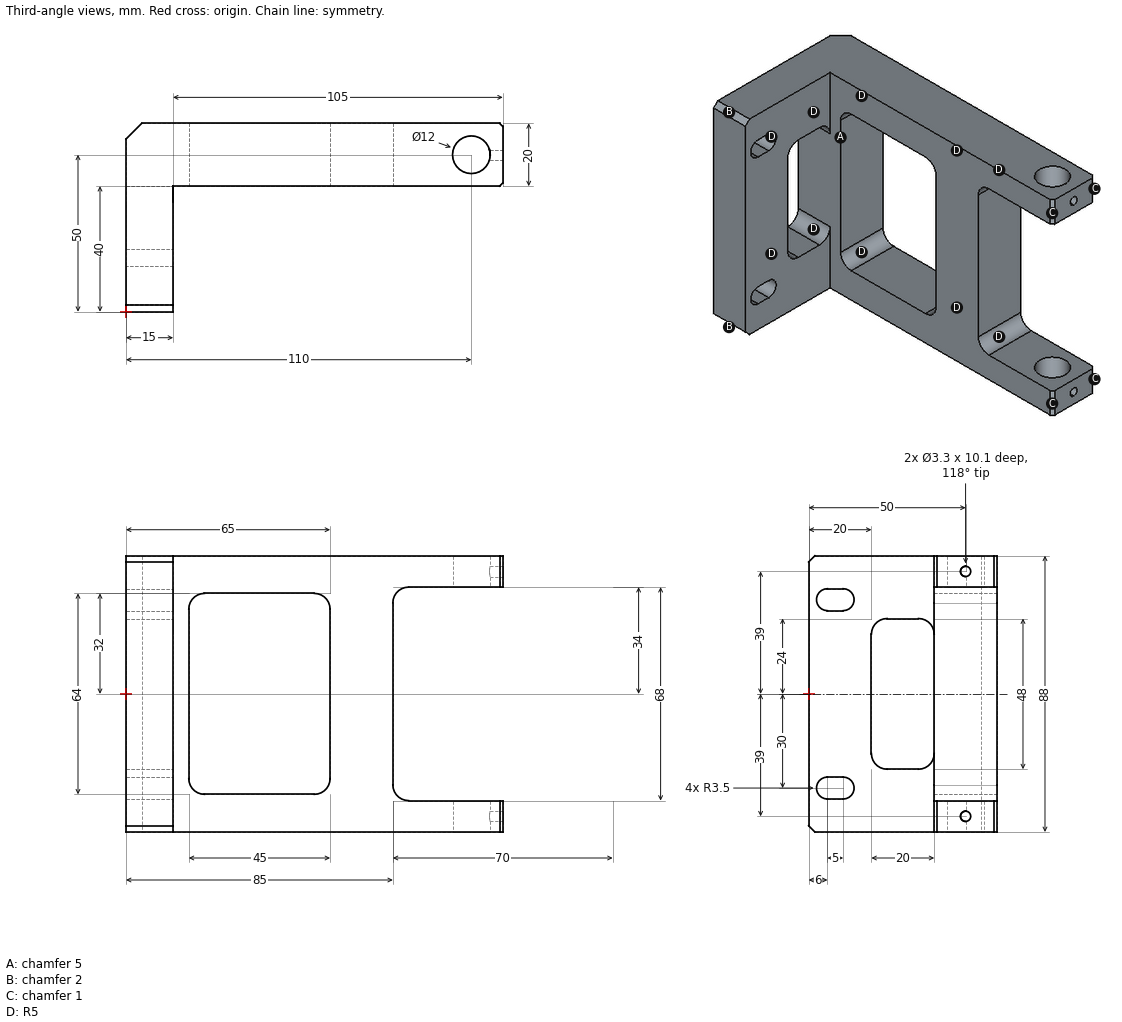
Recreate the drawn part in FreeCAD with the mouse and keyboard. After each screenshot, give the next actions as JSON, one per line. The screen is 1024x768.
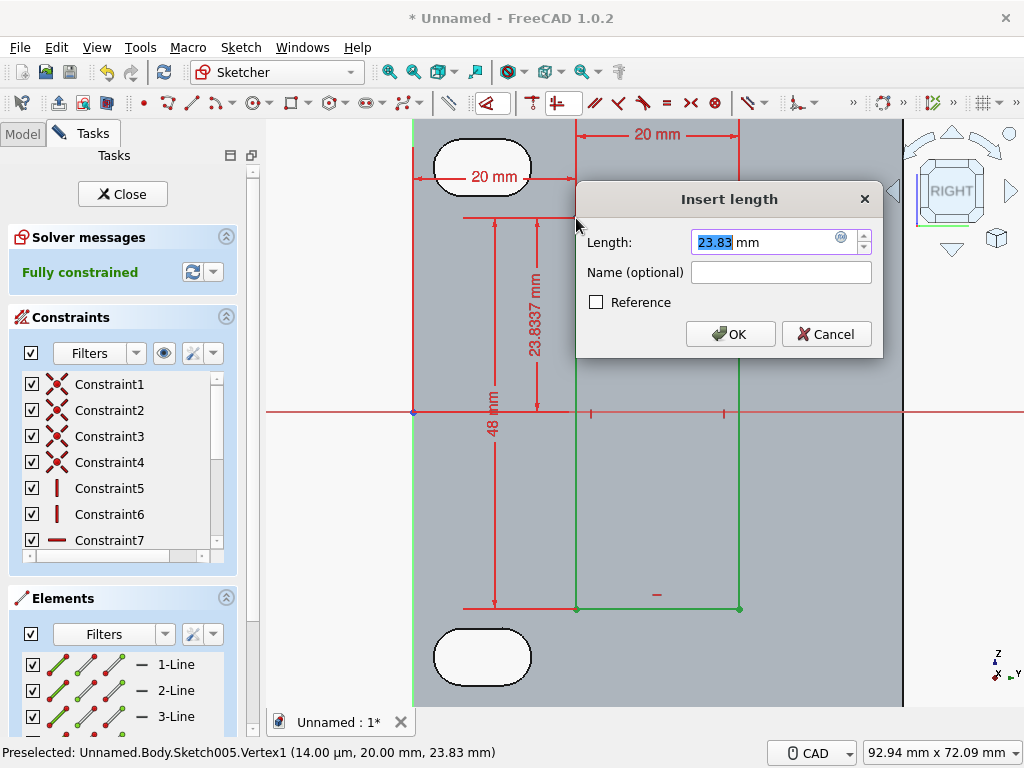
{"action": "type", "text": "24"}
{"action": "key", "text": "Return"}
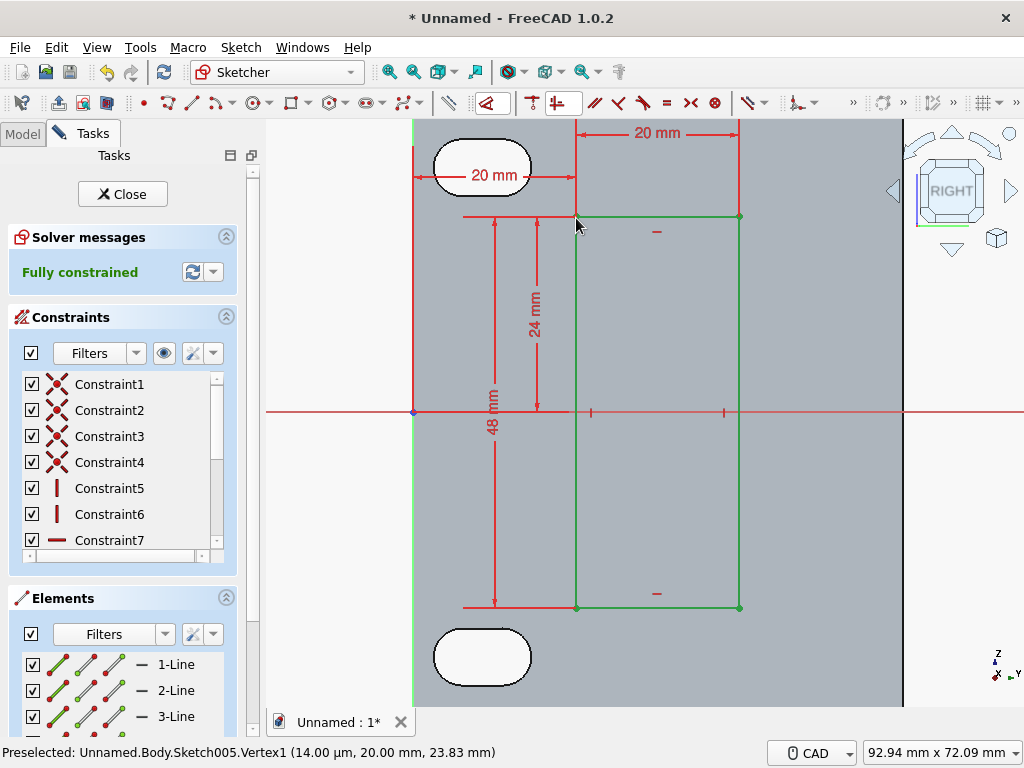
{"action": "left_click", "coordinate": [123, 194]}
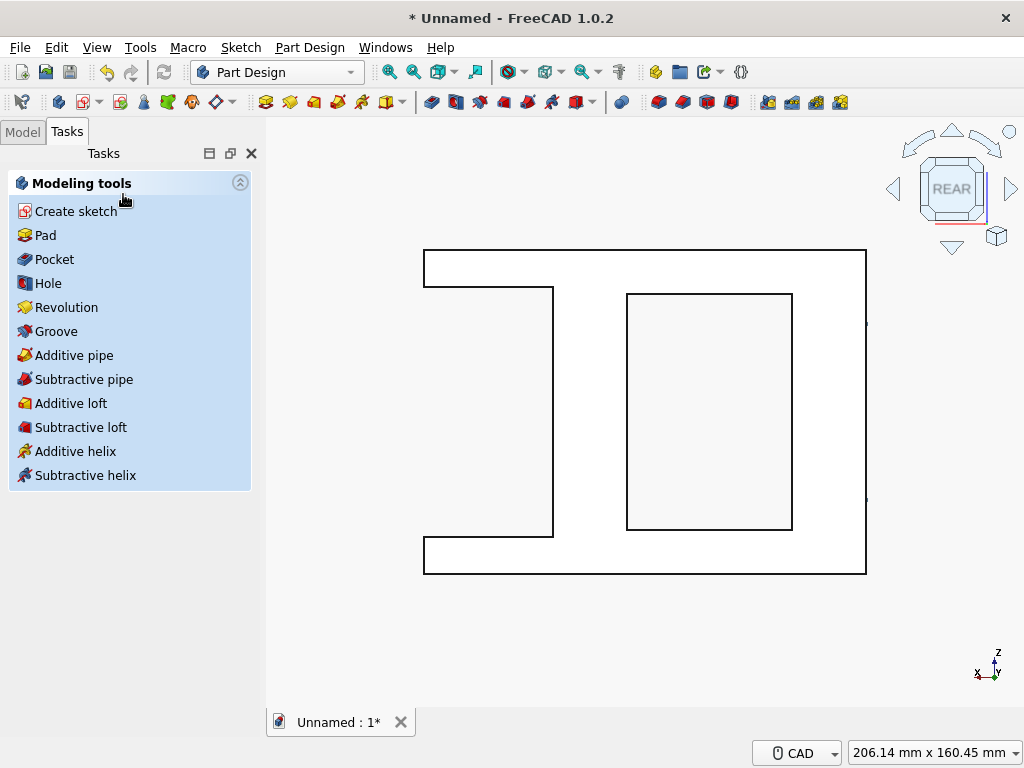
{"action": "left_click", "coordinate": [432, 102]}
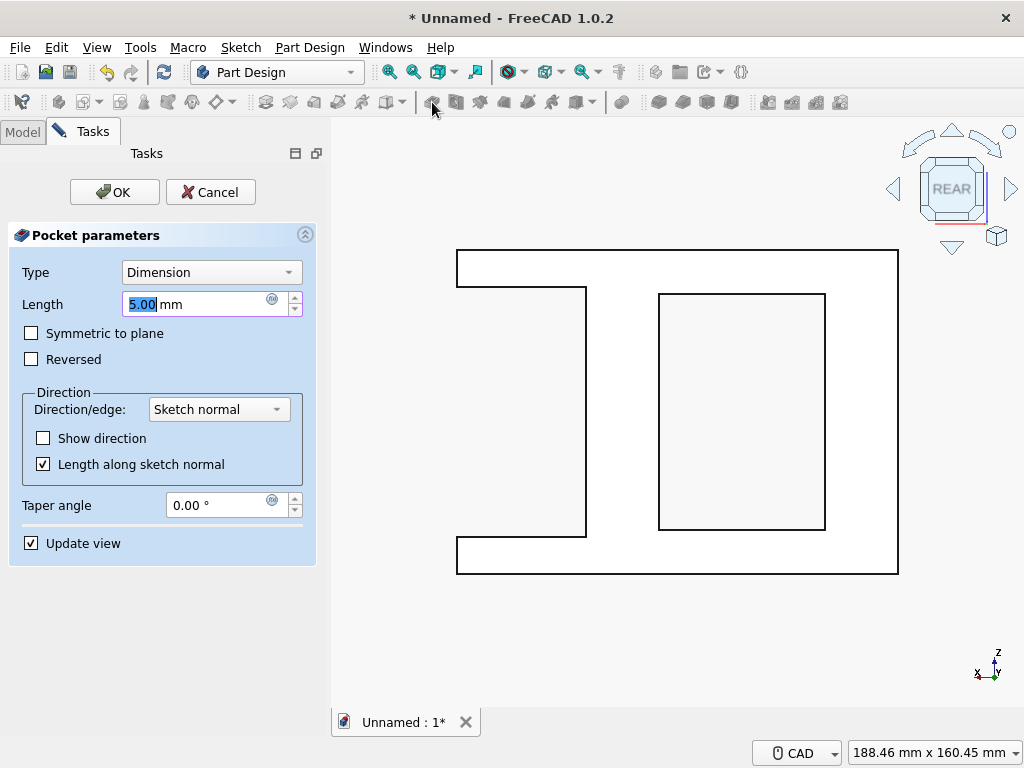
{"action": "left_click", "coordinate": [212, 272]}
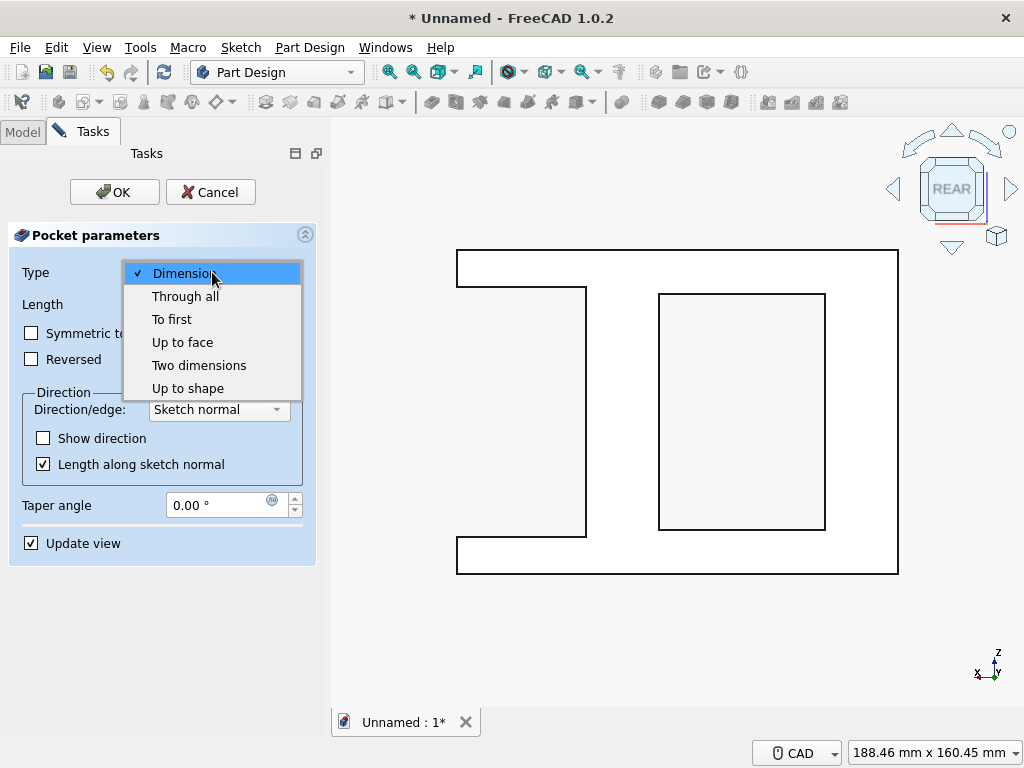
{"action": "left_click", "coordinate": [212, 296]}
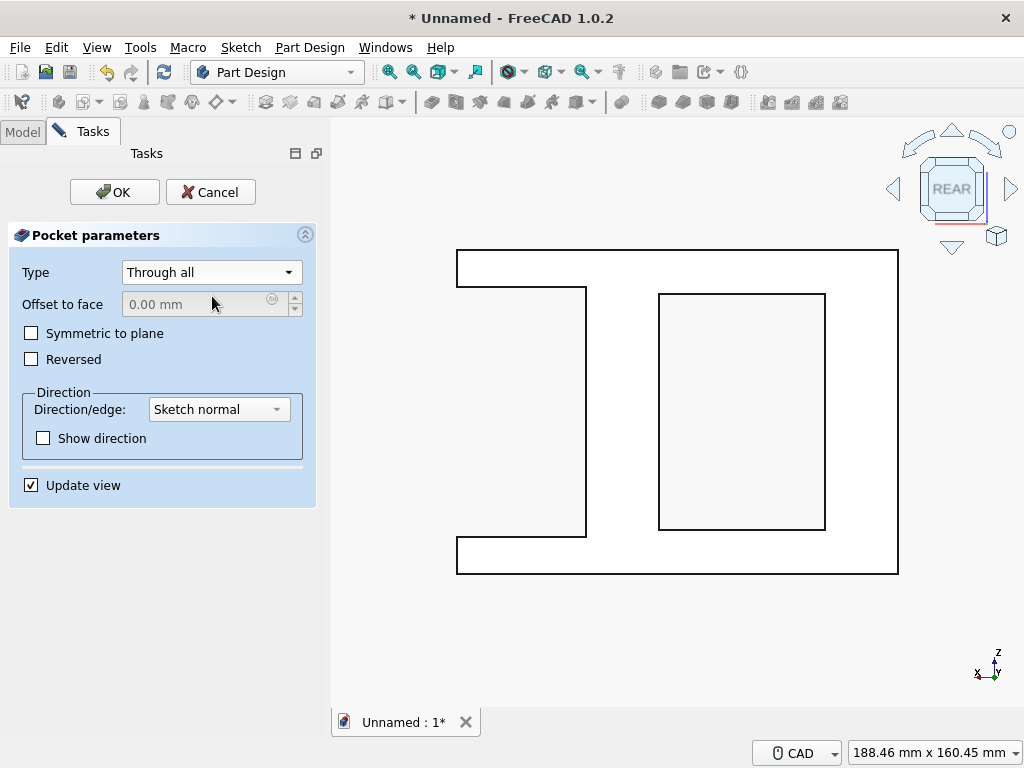
{"action": "left_click", "coordinate": [30, 359]}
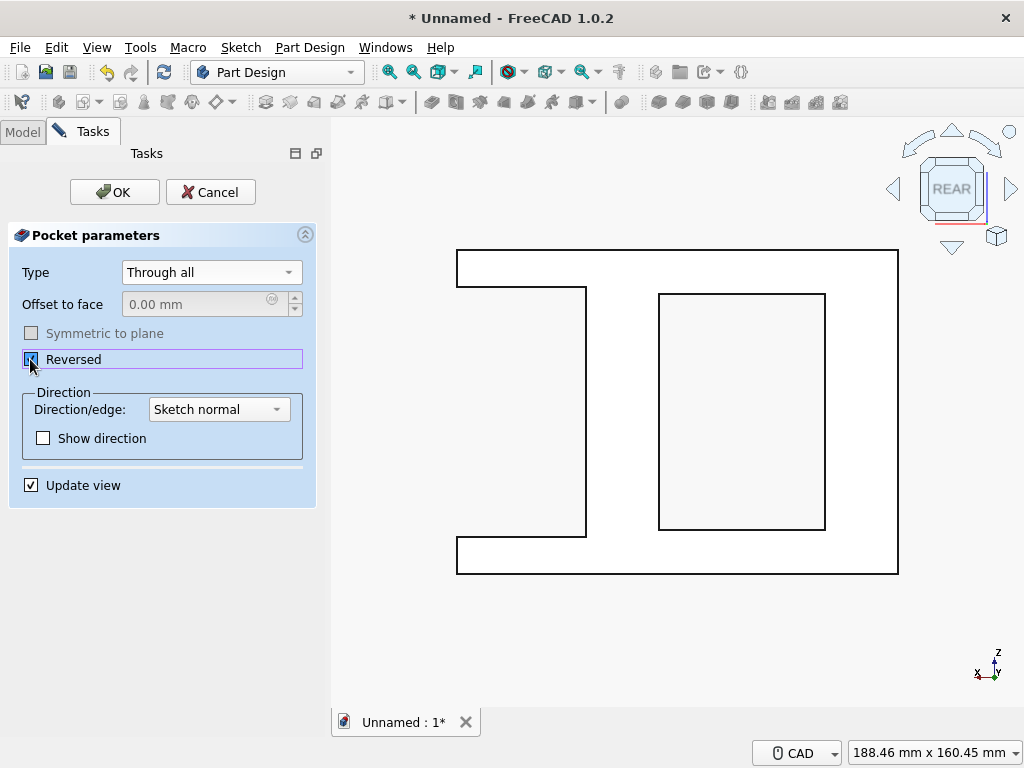
{"action": "left_click", "coordinate": [115, 192]}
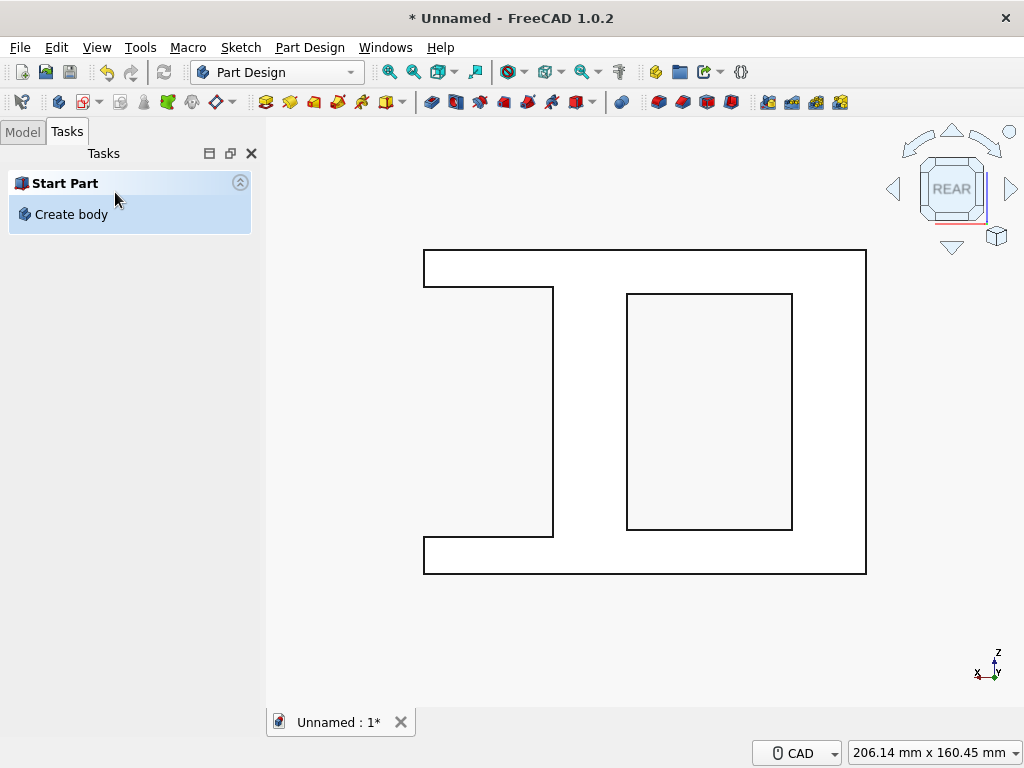
{"action": "left_click", "coordinate": [866, 411]}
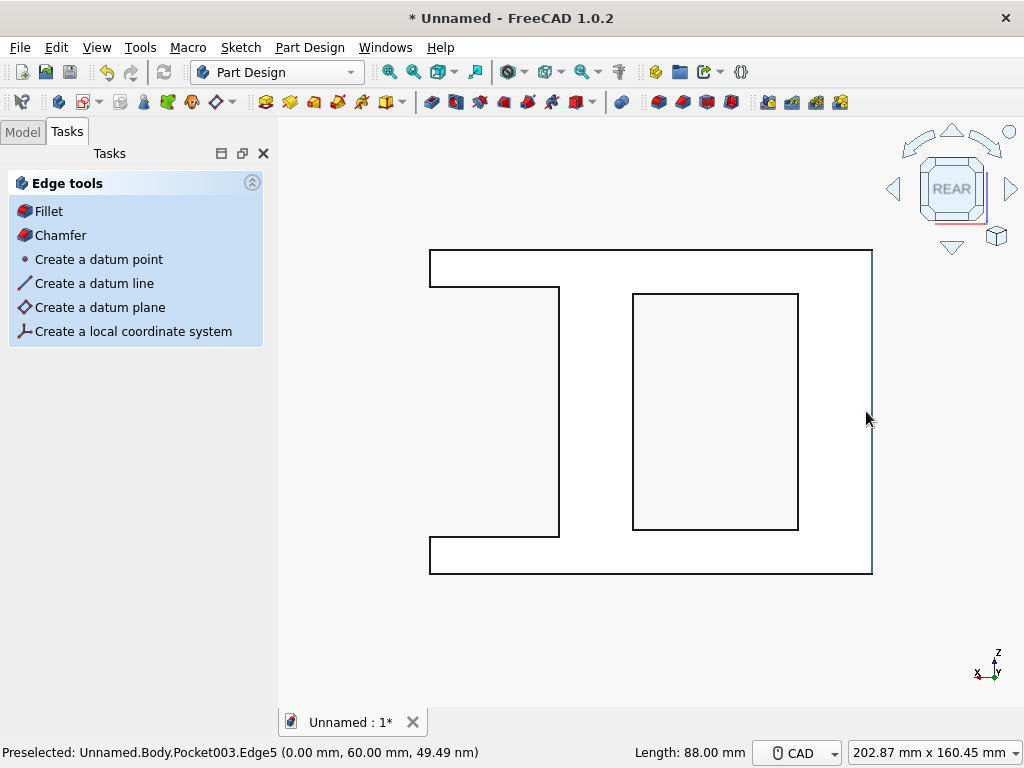
{"action": "left_click", "coordinate": [684, 102]}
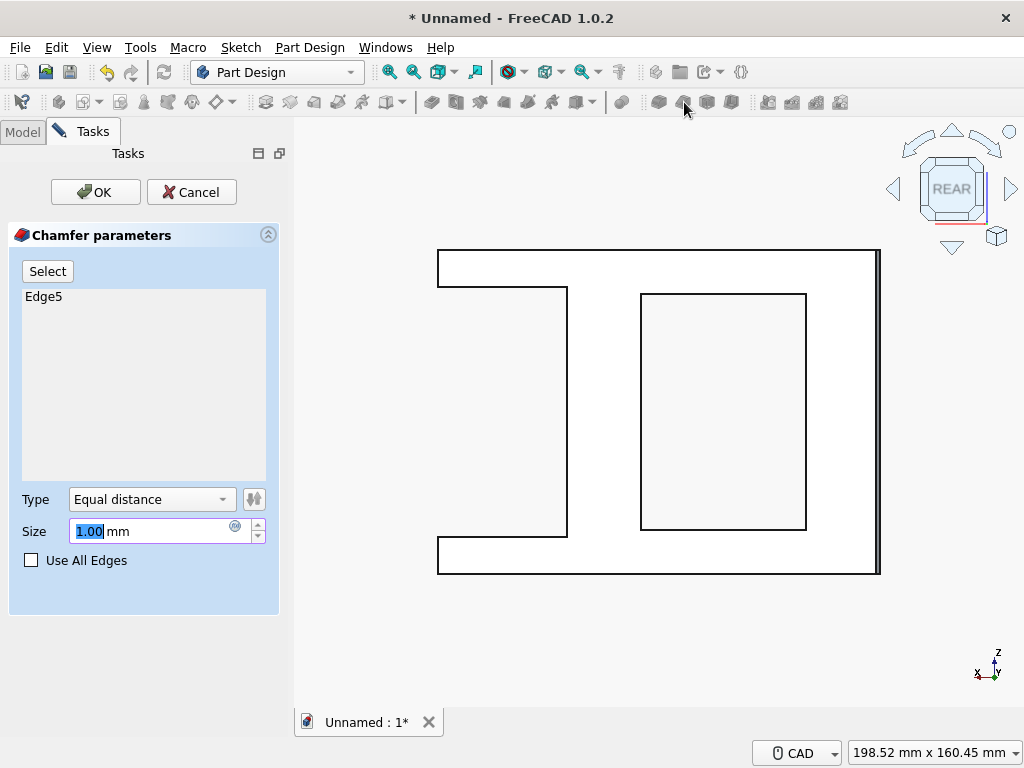
{"action": "type", "text": "5"}
{"action": "key", "text": "Tab"}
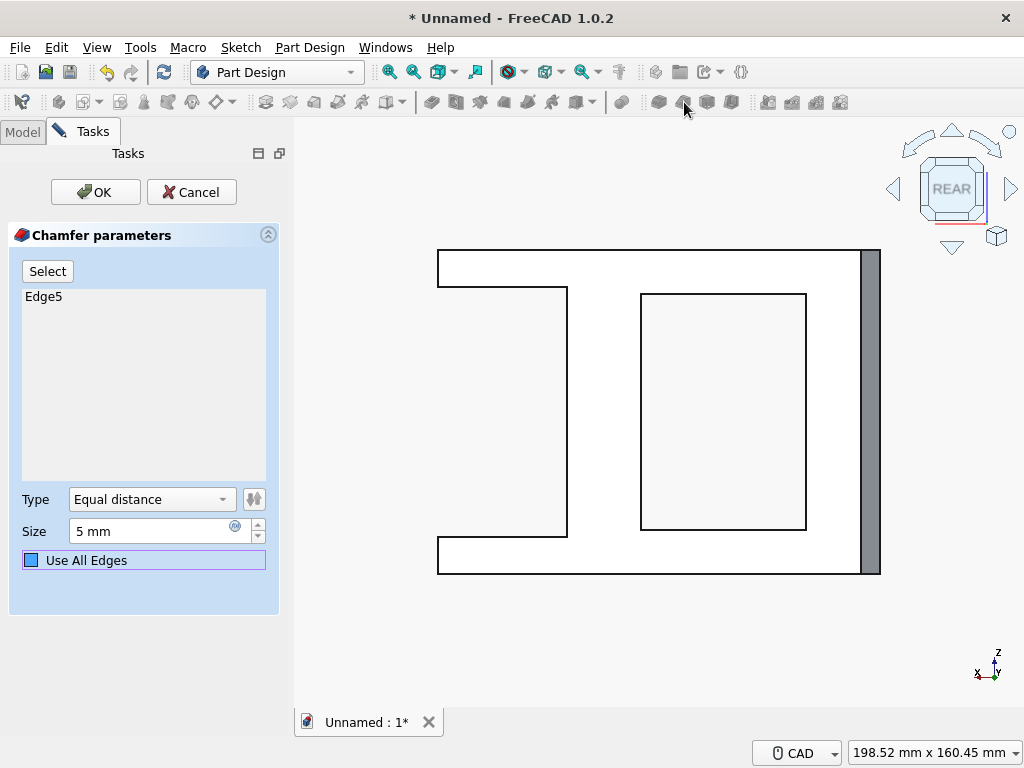
{"action": "left_click", "coordinate": [96, 192]}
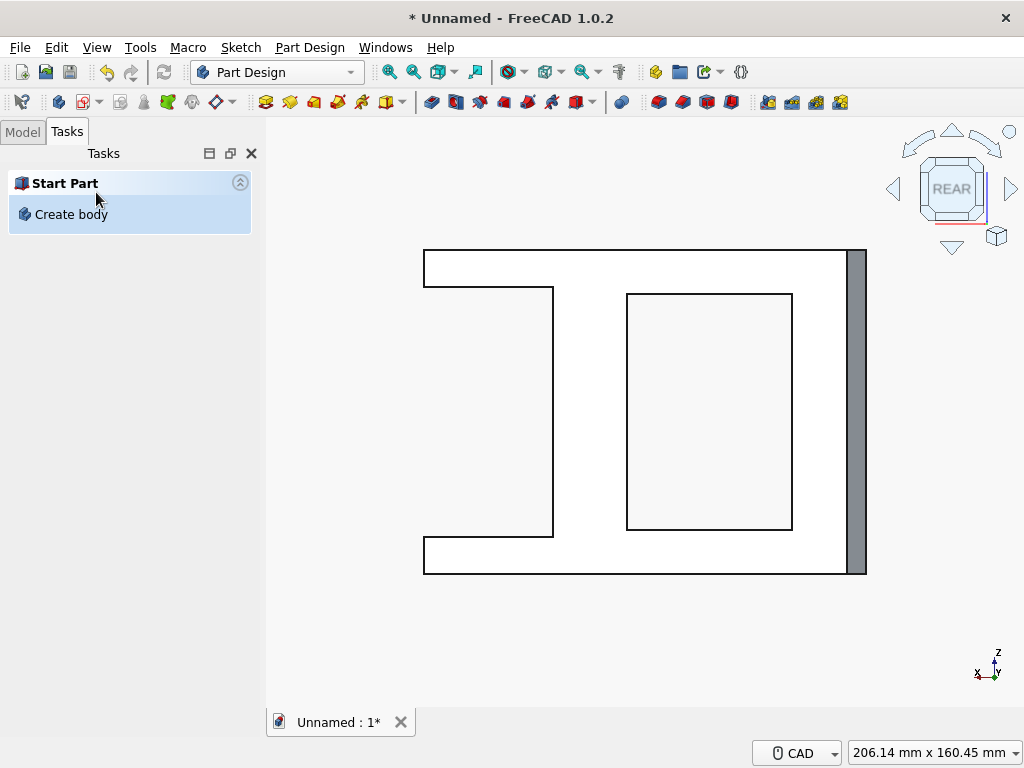
{"action": "key", "text": "0"}